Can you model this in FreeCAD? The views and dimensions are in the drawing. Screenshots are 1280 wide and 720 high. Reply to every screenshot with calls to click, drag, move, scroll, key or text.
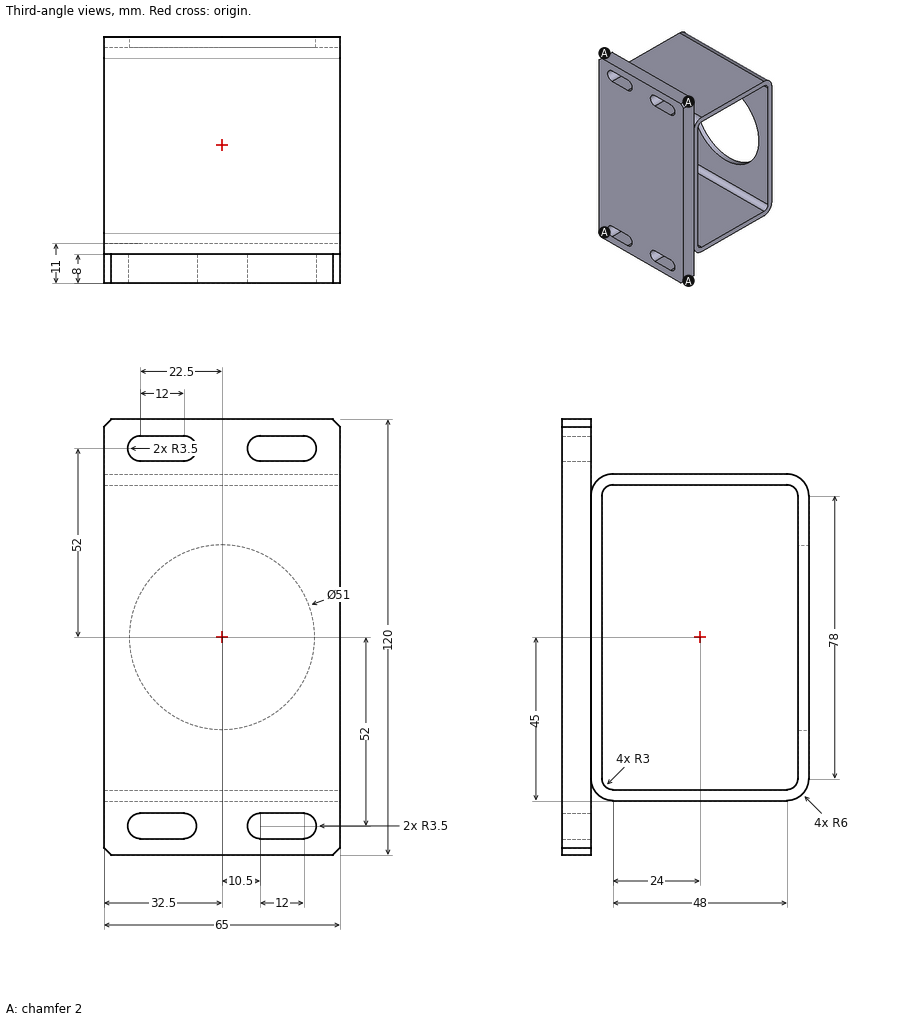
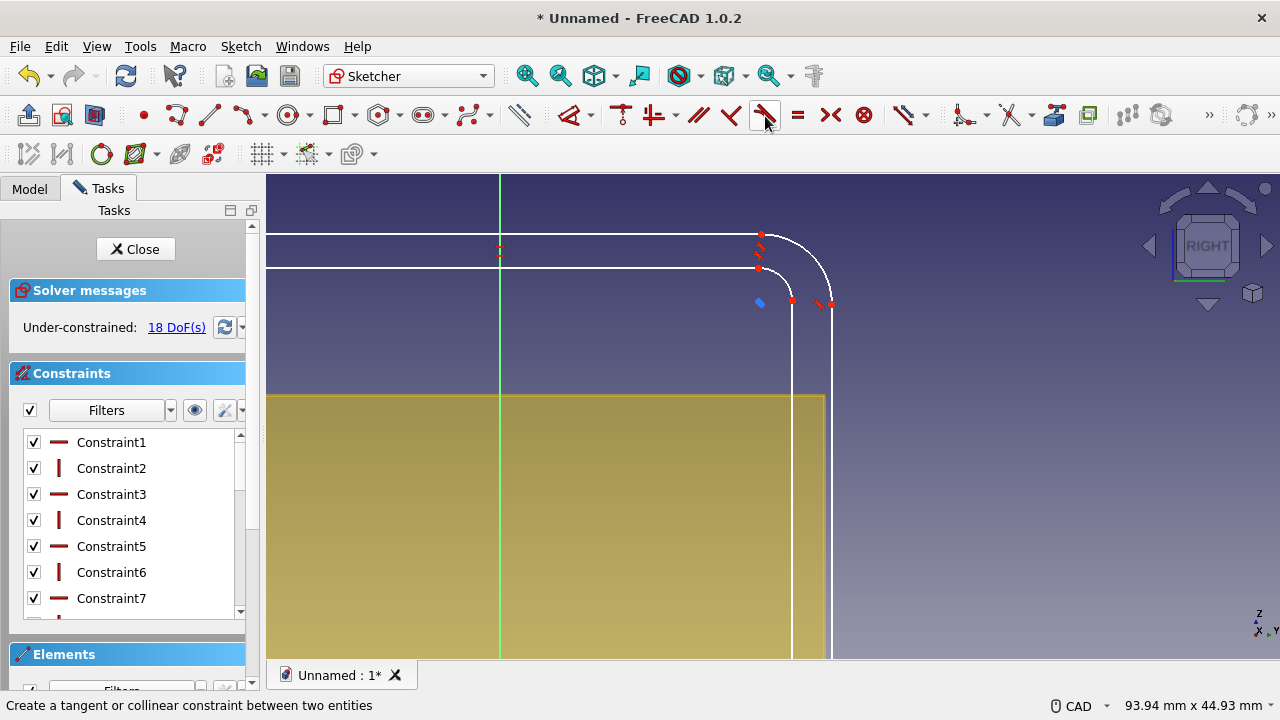
click(792, 554)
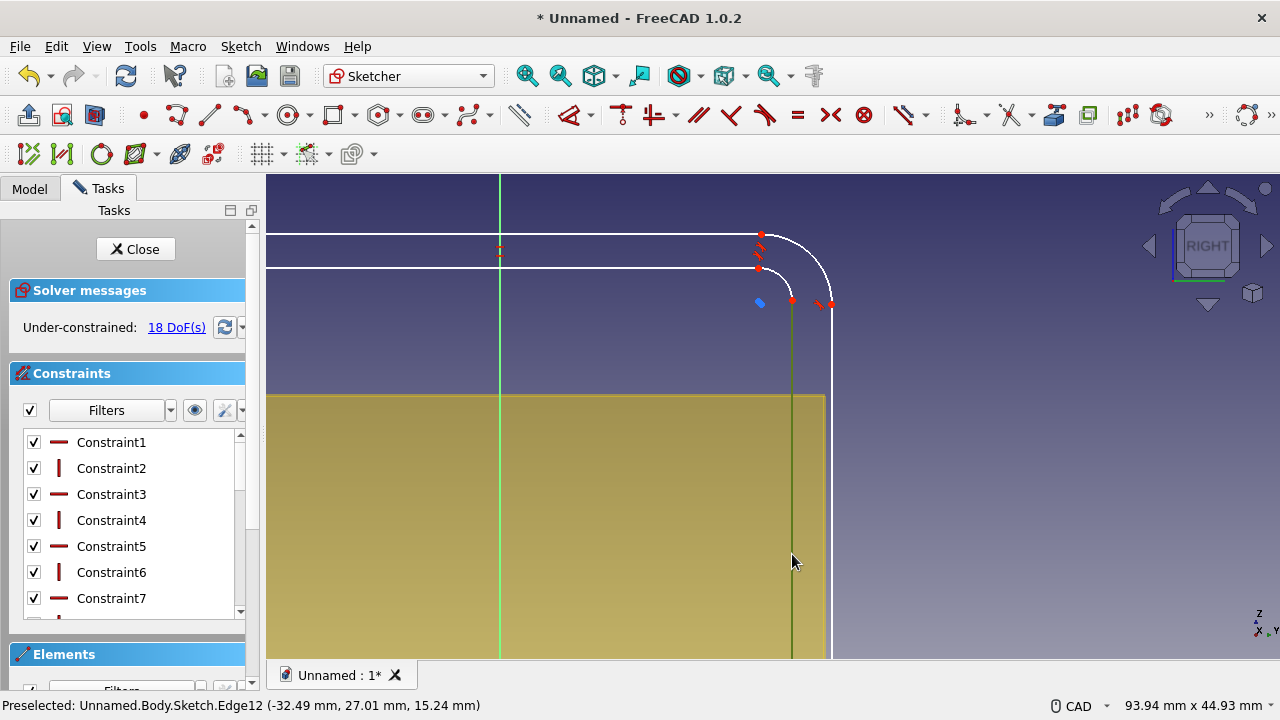
click(788, 286)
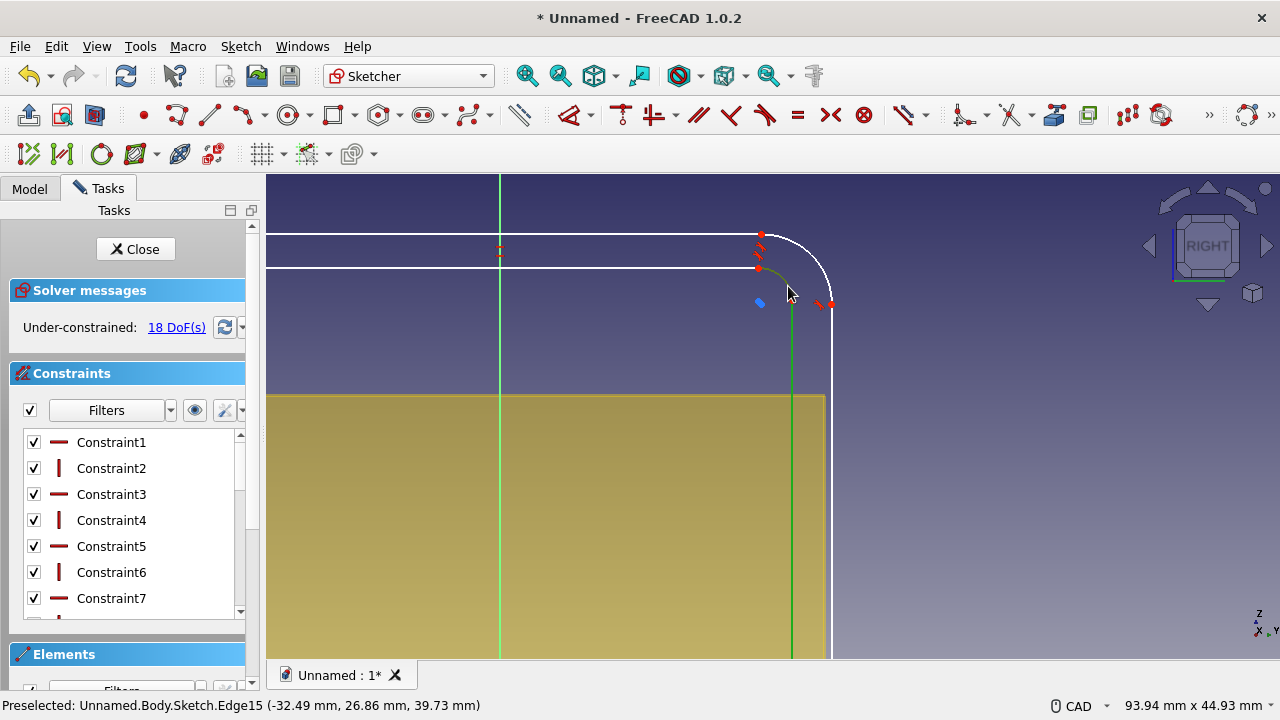
click(765, 116)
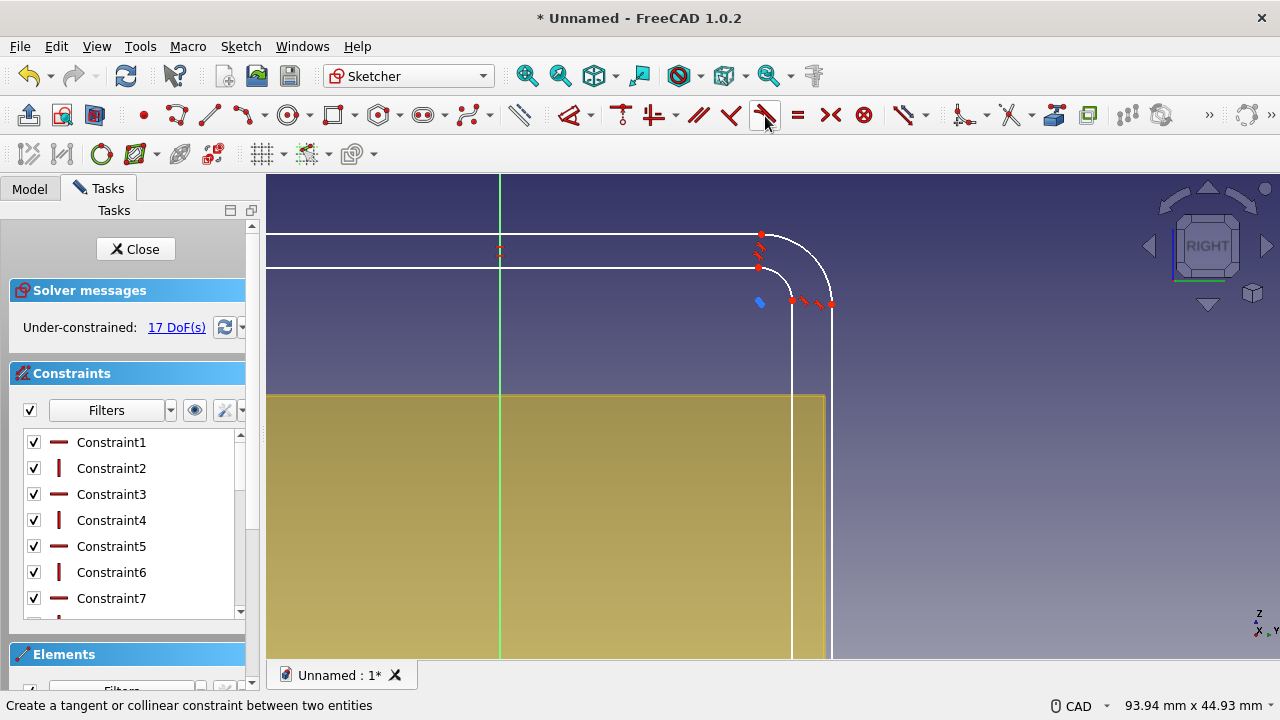
click(792, 554)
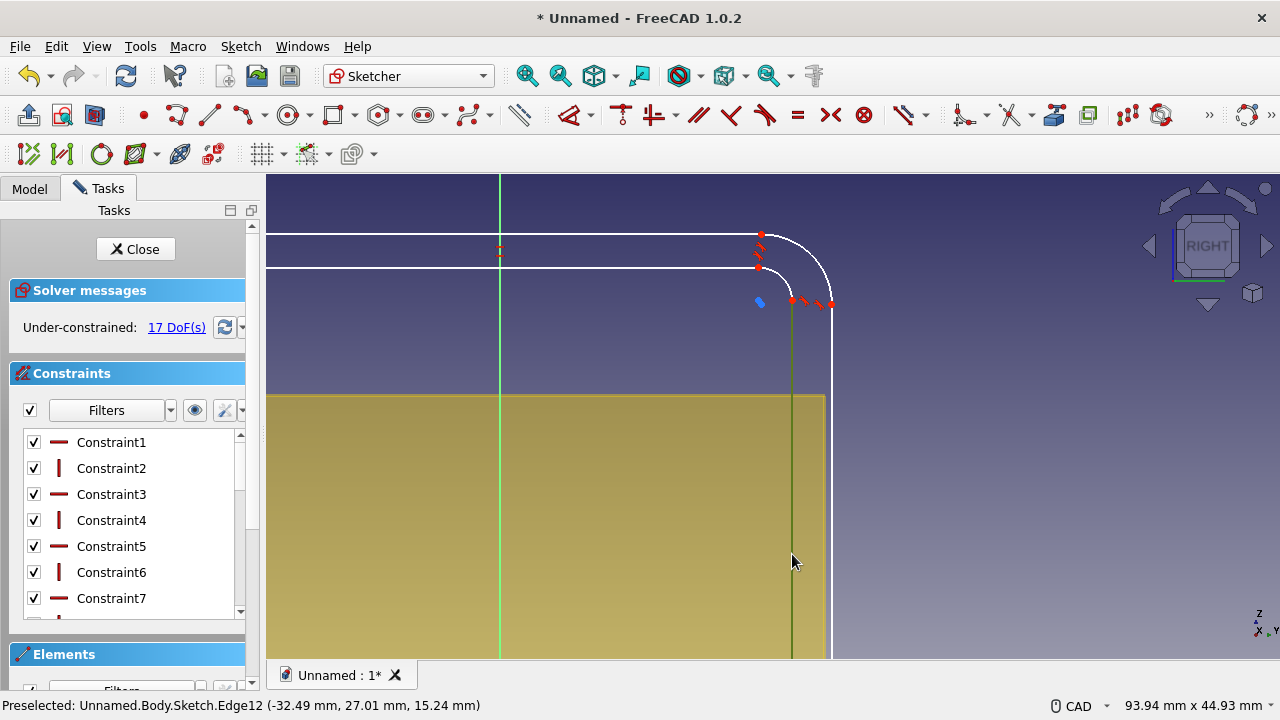
scroll(792, 286, down, 6)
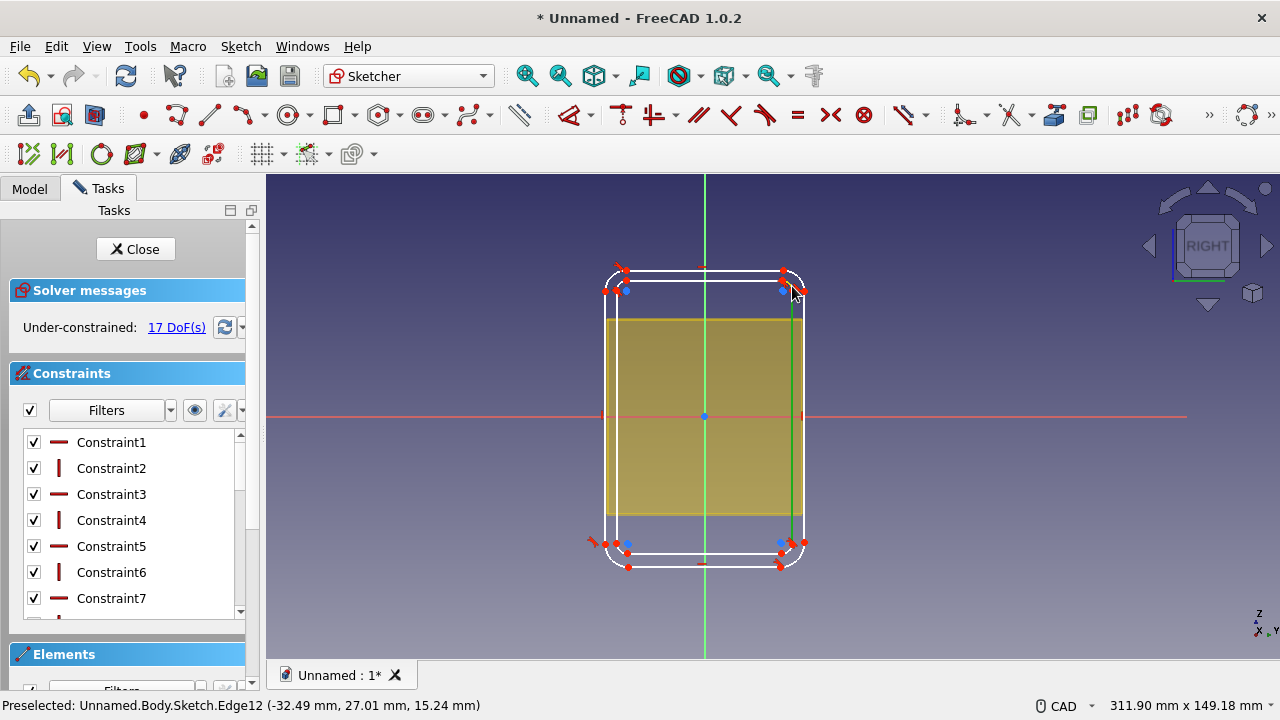
scroll(786, 553, up, 6)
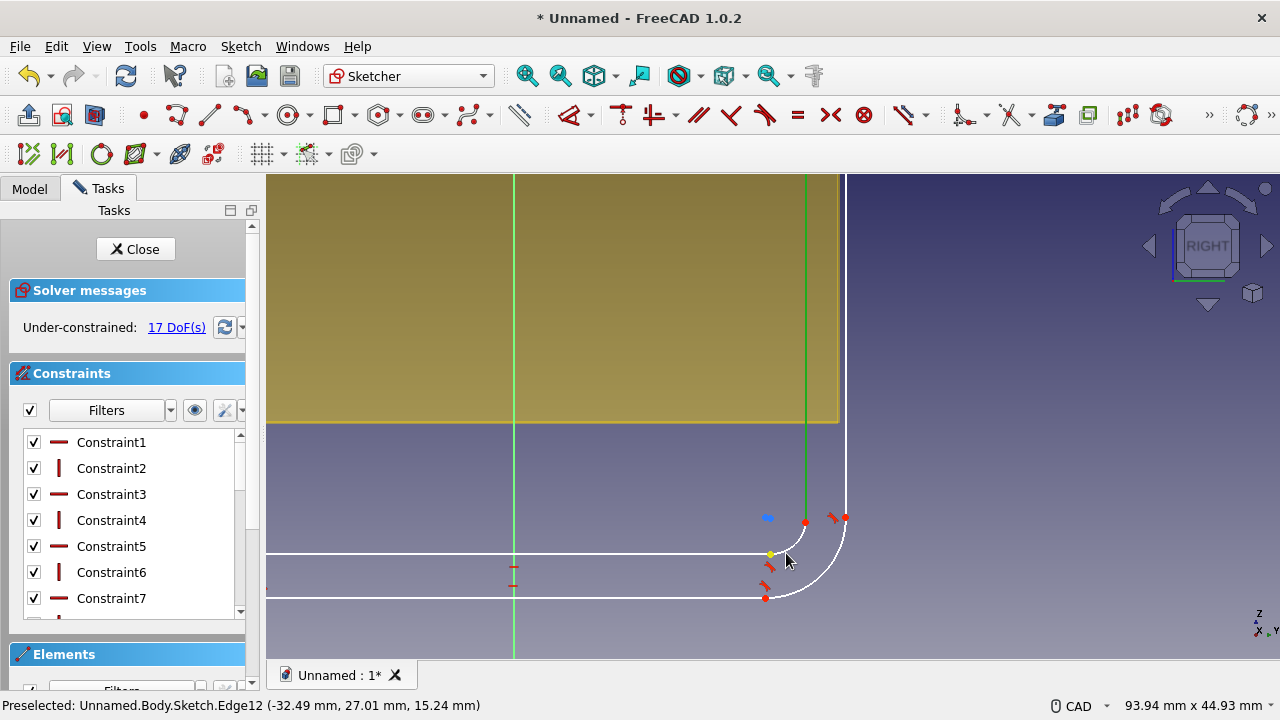
click(786, 551)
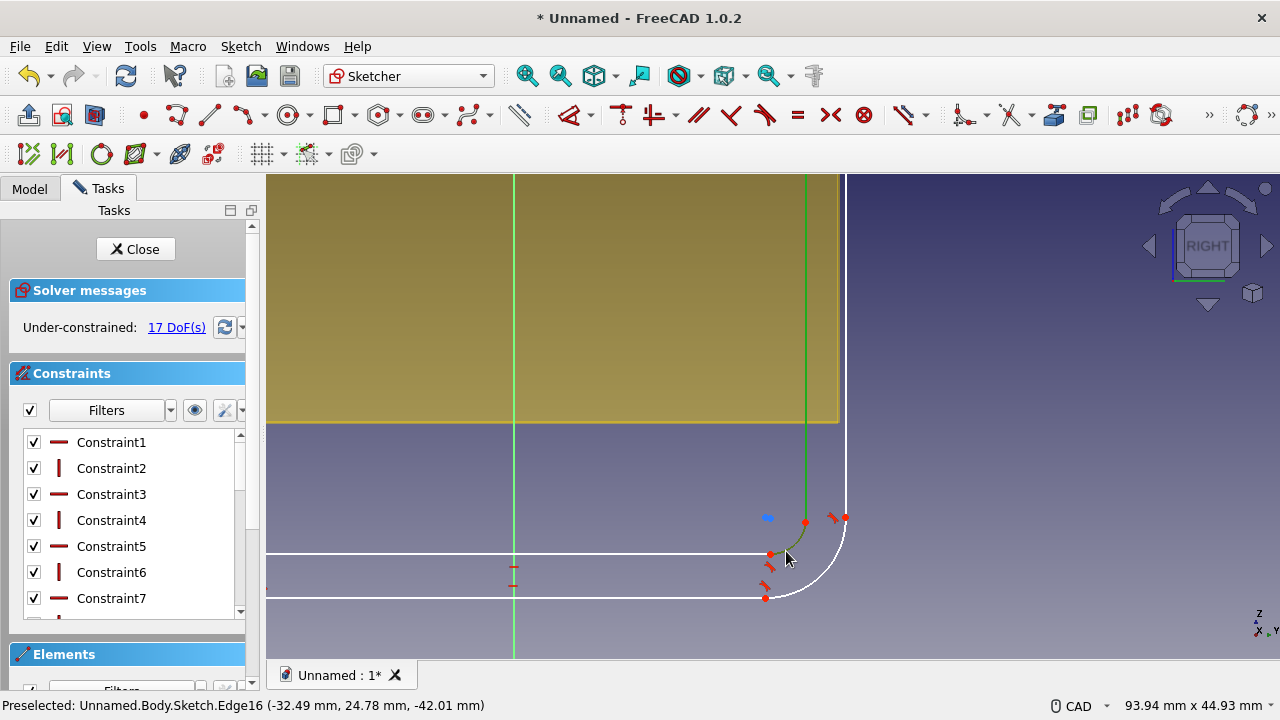
click(765, 116)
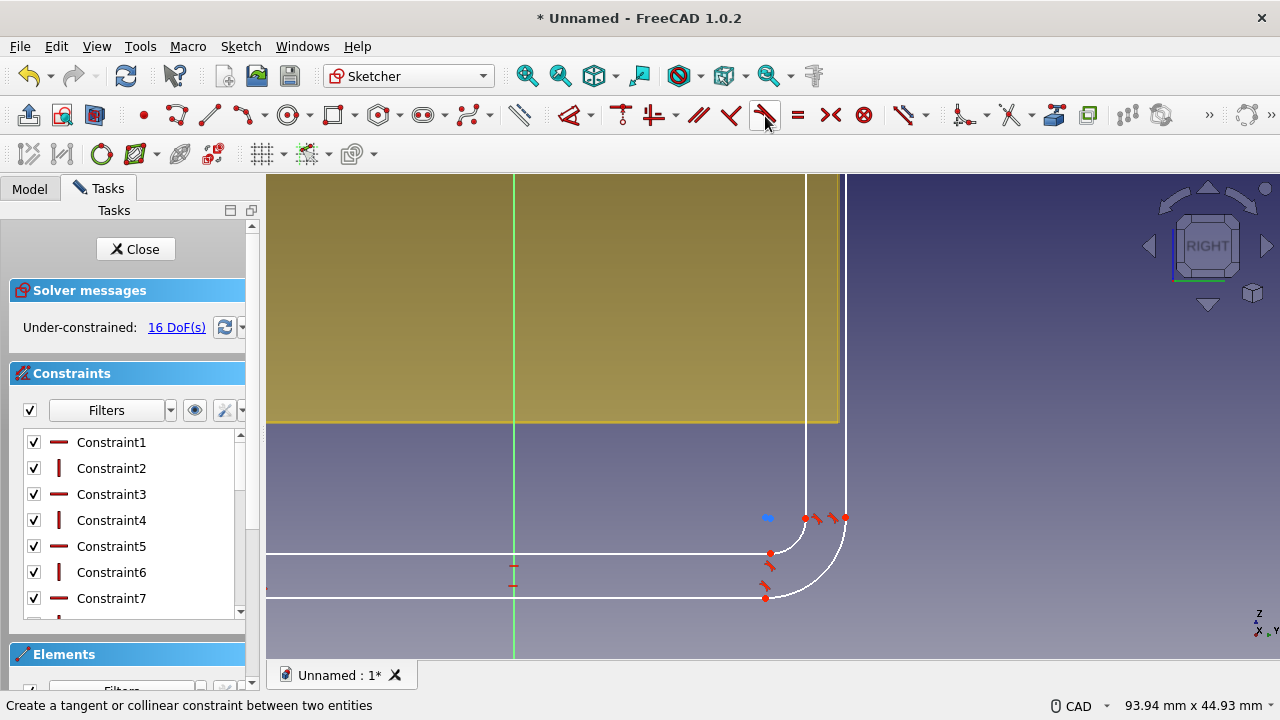
scroll(786, 553, down, 6)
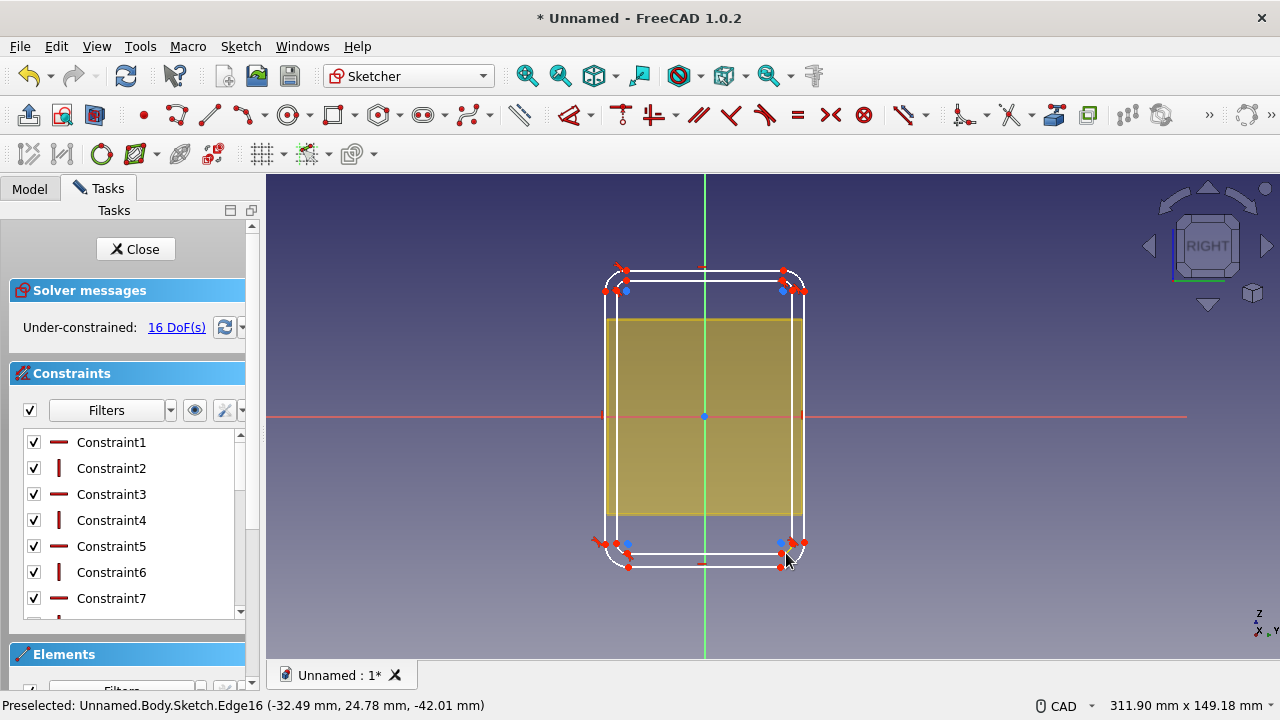
scroll(608, 555, up, 2)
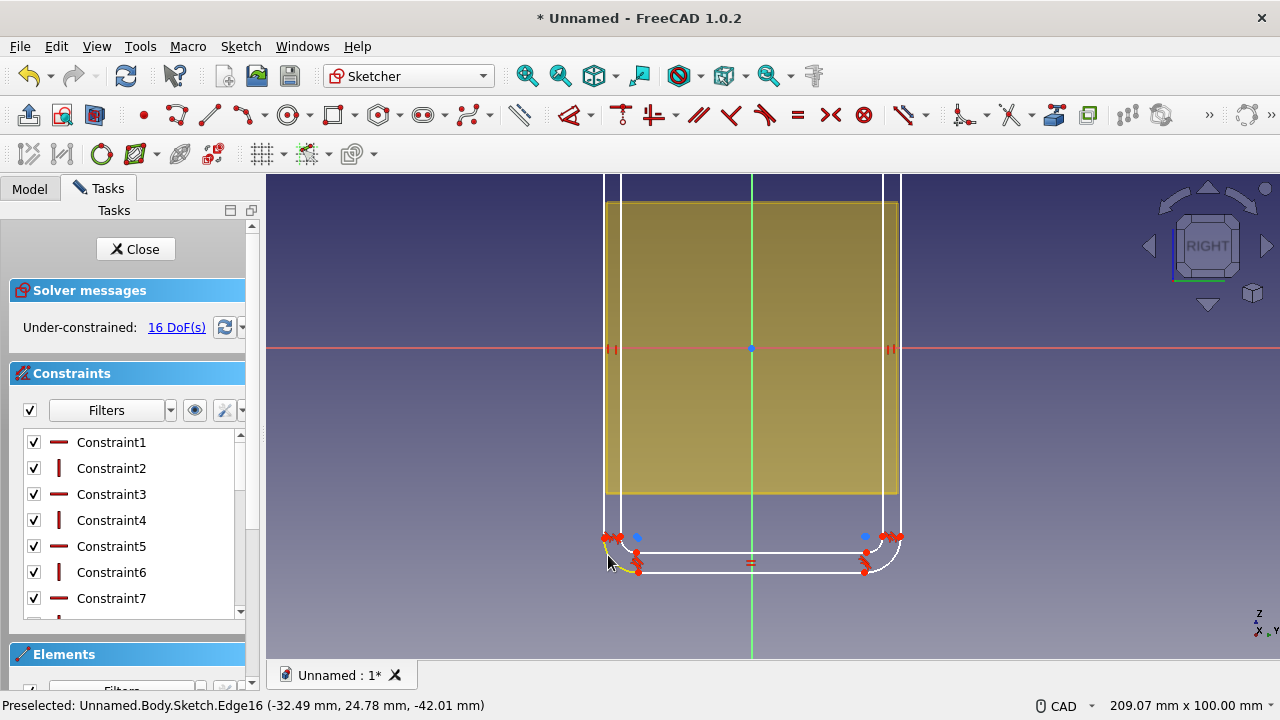
click(608, 554)